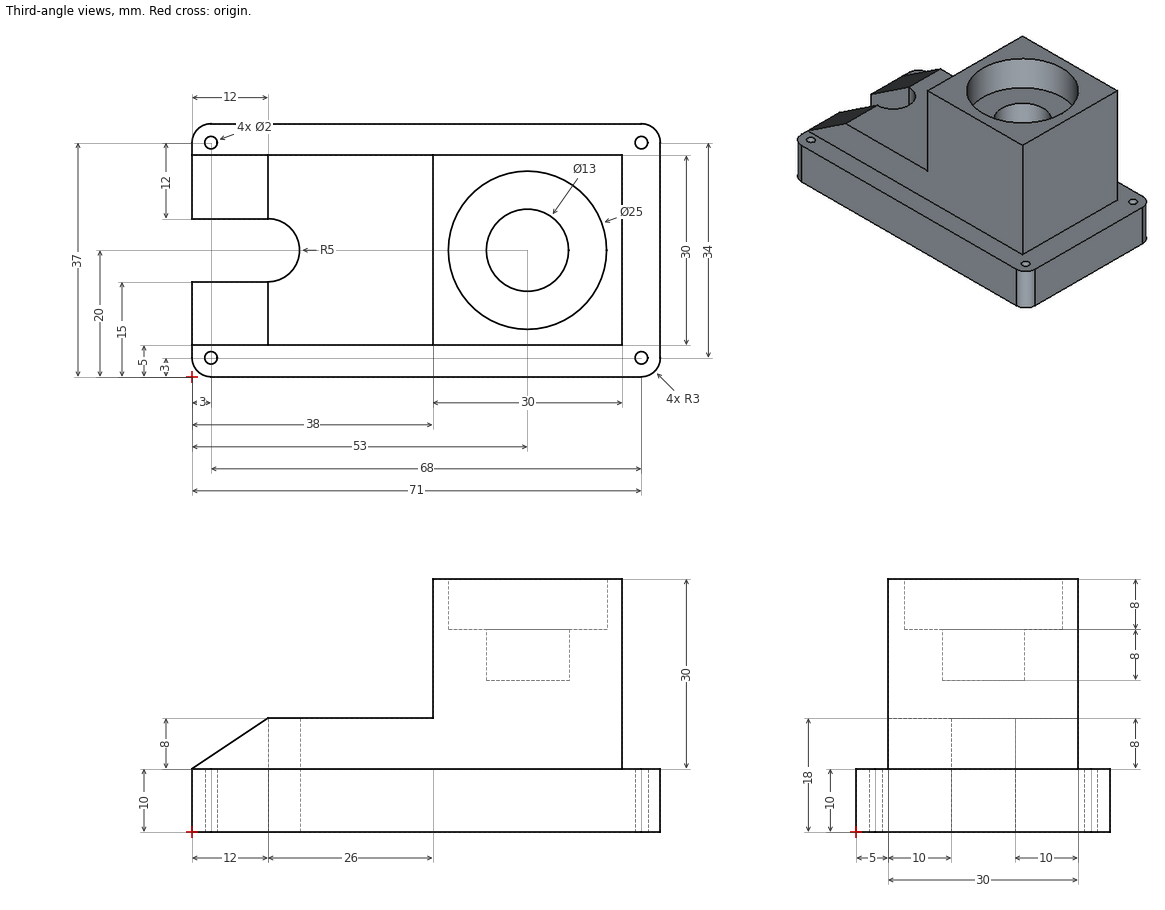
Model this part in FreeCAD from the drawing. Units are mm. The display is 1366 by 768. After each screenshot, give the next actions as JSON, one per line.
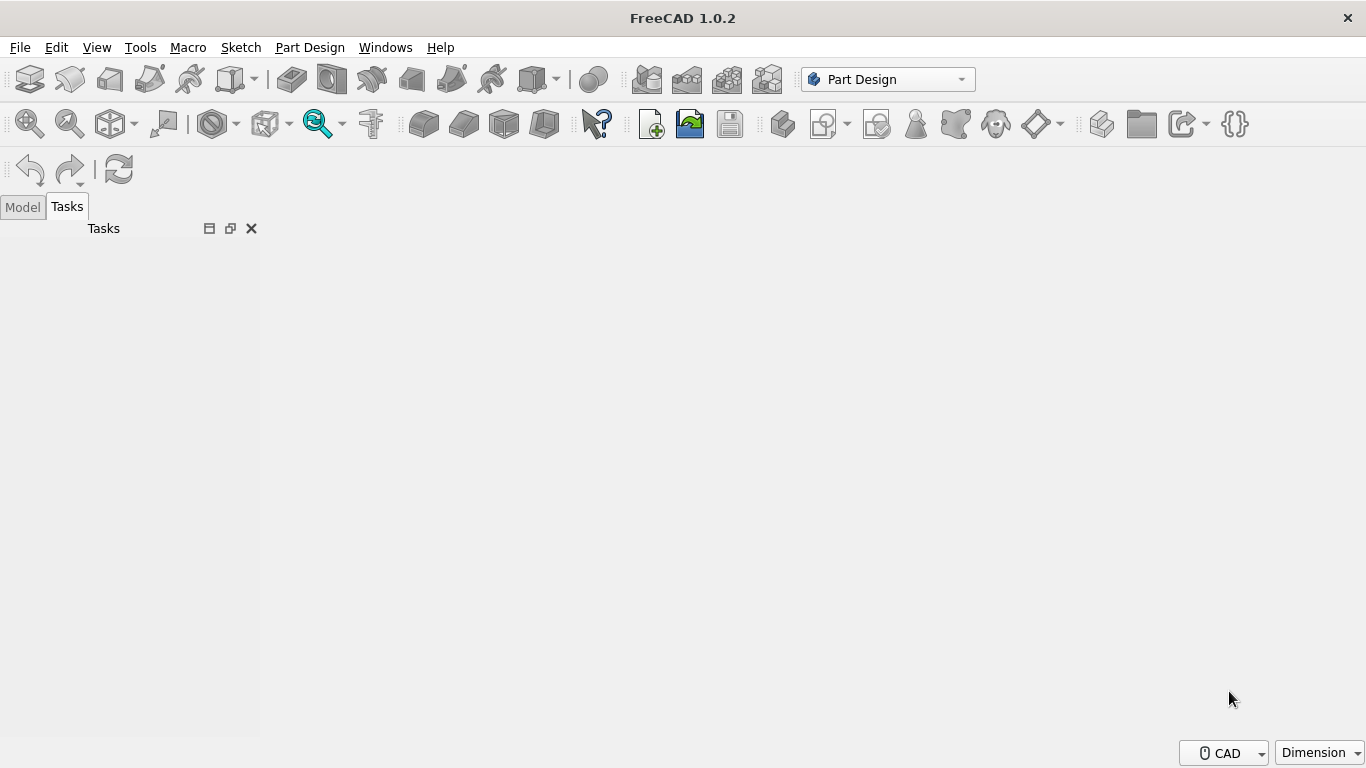
{"action": "left_click", "coordinate": [650, 124]}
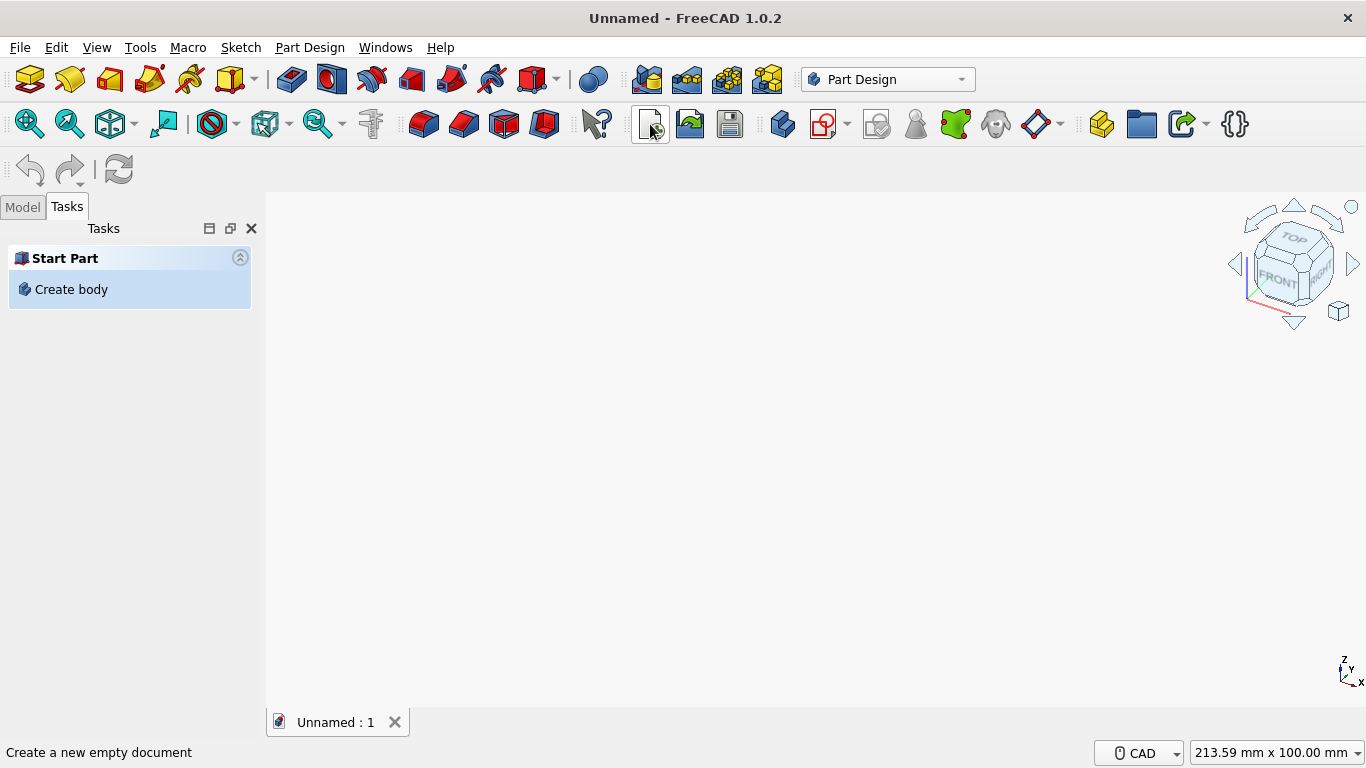
{"action": "left_click", "coordinate": [824, 124]}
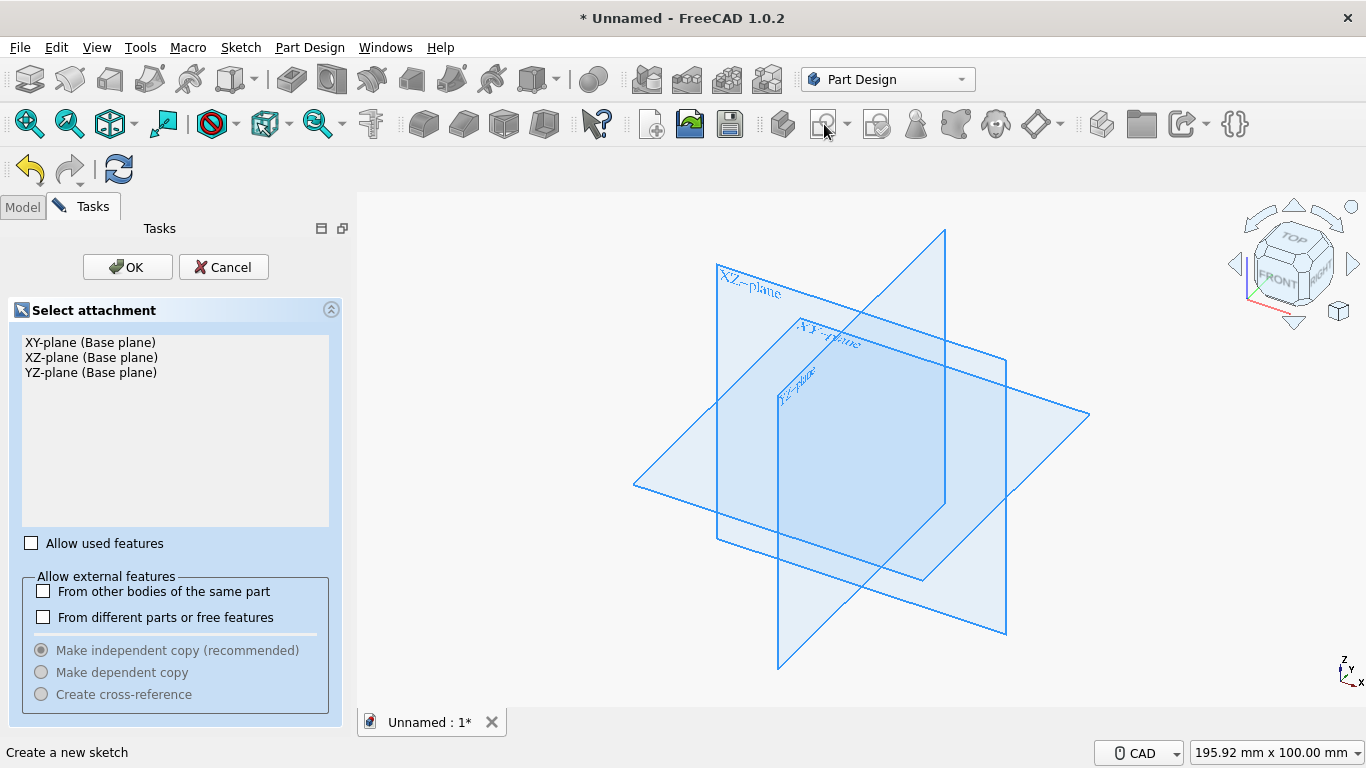
{"action": "left_click", "coordinate": [82, 342]}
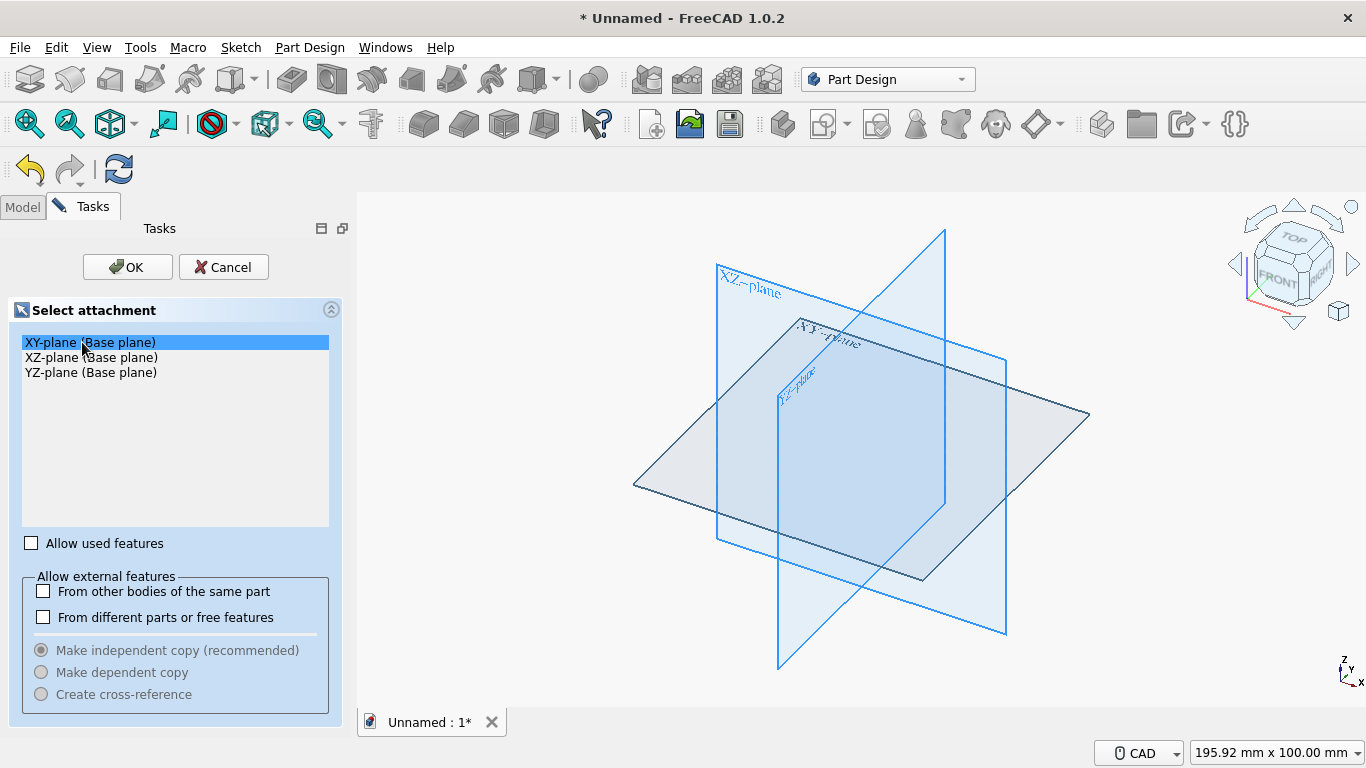
{"action": "left_click", "coordinate": [128, 267]}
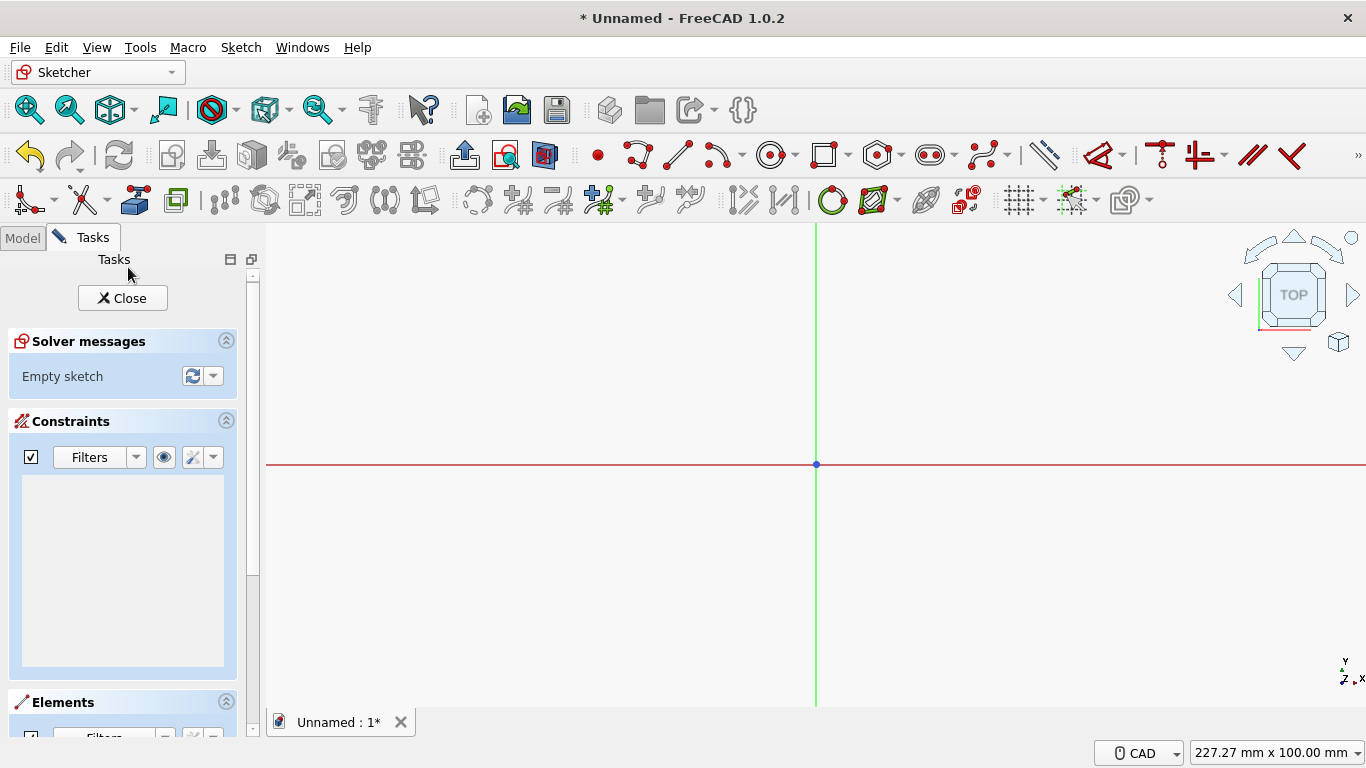
{"action": "scroll", "coordinate": [1201, 251], "scroll_direction": "up", "scroll_amount": 2}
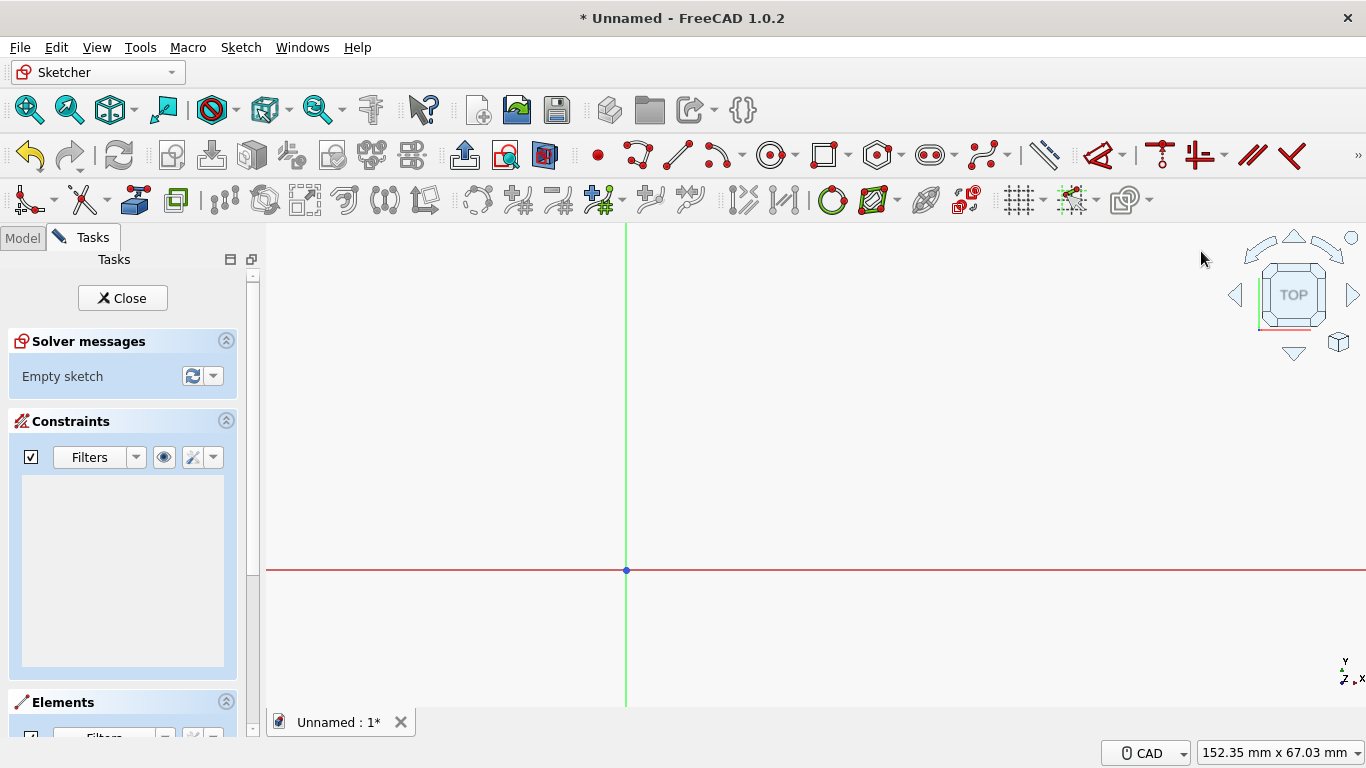
{"action": "left_click", "coordinate": [678, 156]}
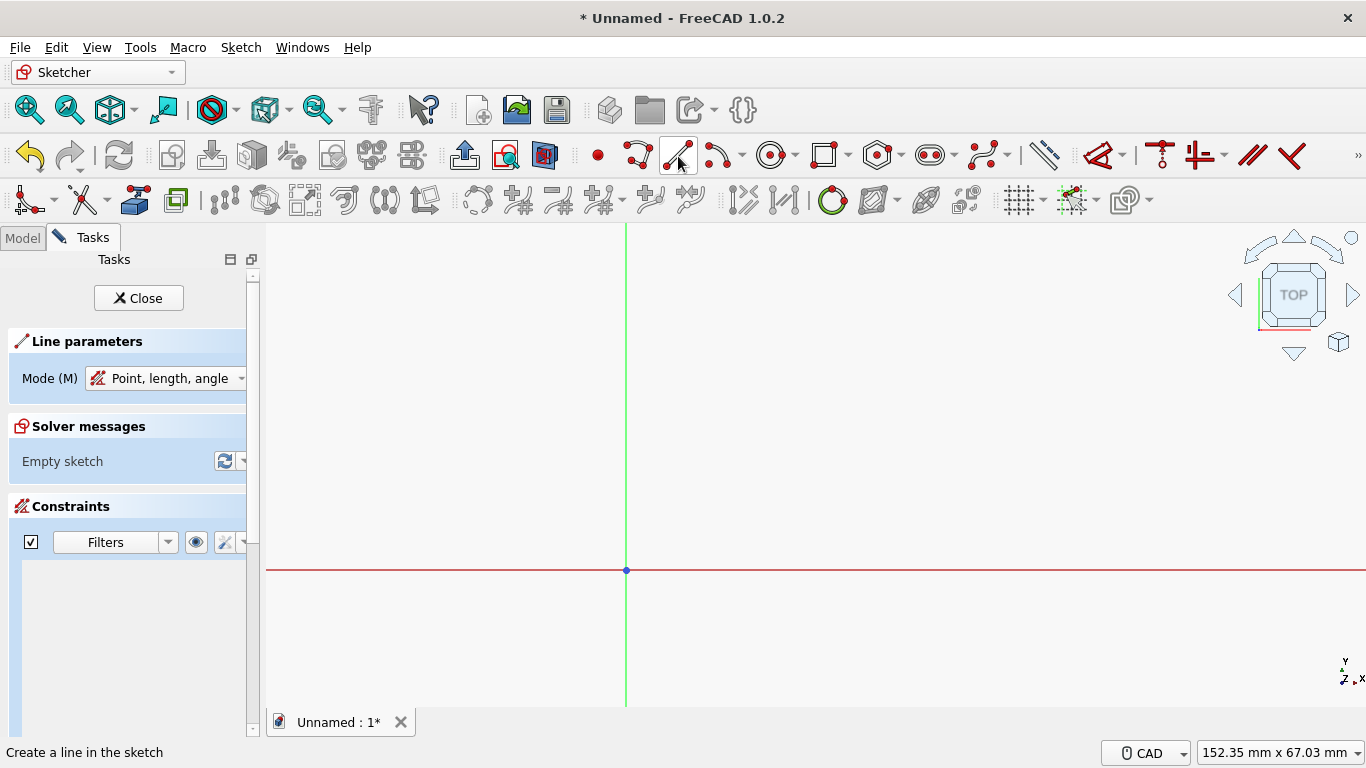
{"action": "left_click", "coordinate": [648, 570]}
{"action": "left_click", "coordinate": [1139, 561]}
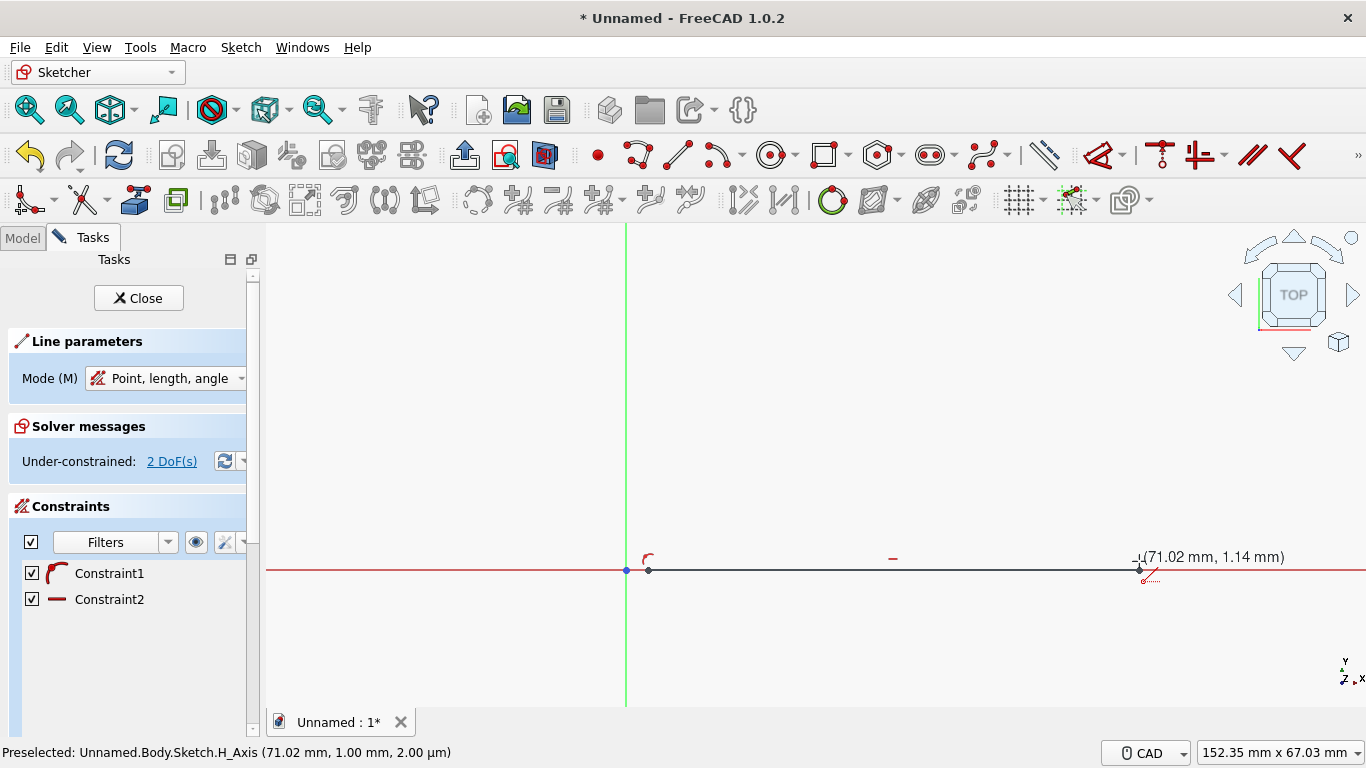
{"action": "left_click", "coordinate": [1161, 549]}
{"action": "left_click", "coordinate": [1161, 303]}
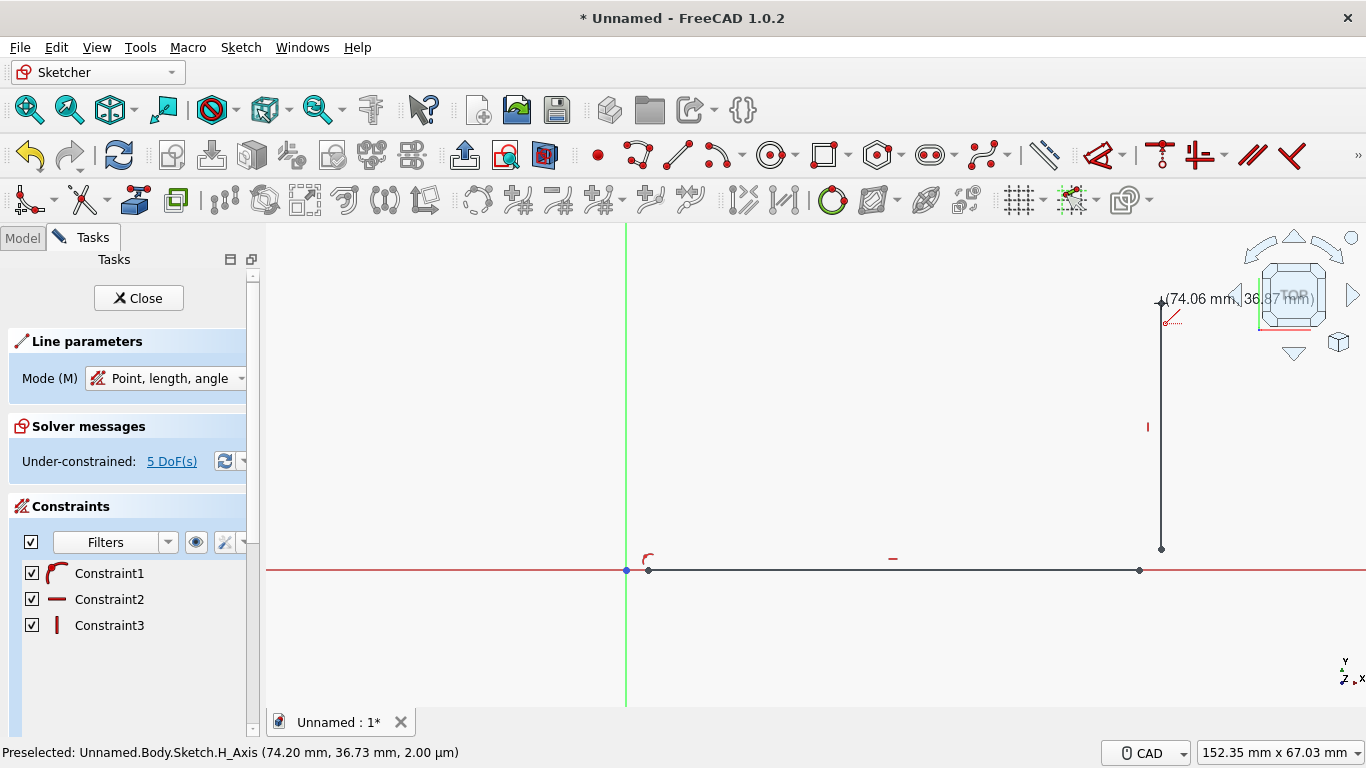
{"action": "left_click", "coordinate": [1139, 281]}
{"action": "left_click", "coordinate": [648, 281]}